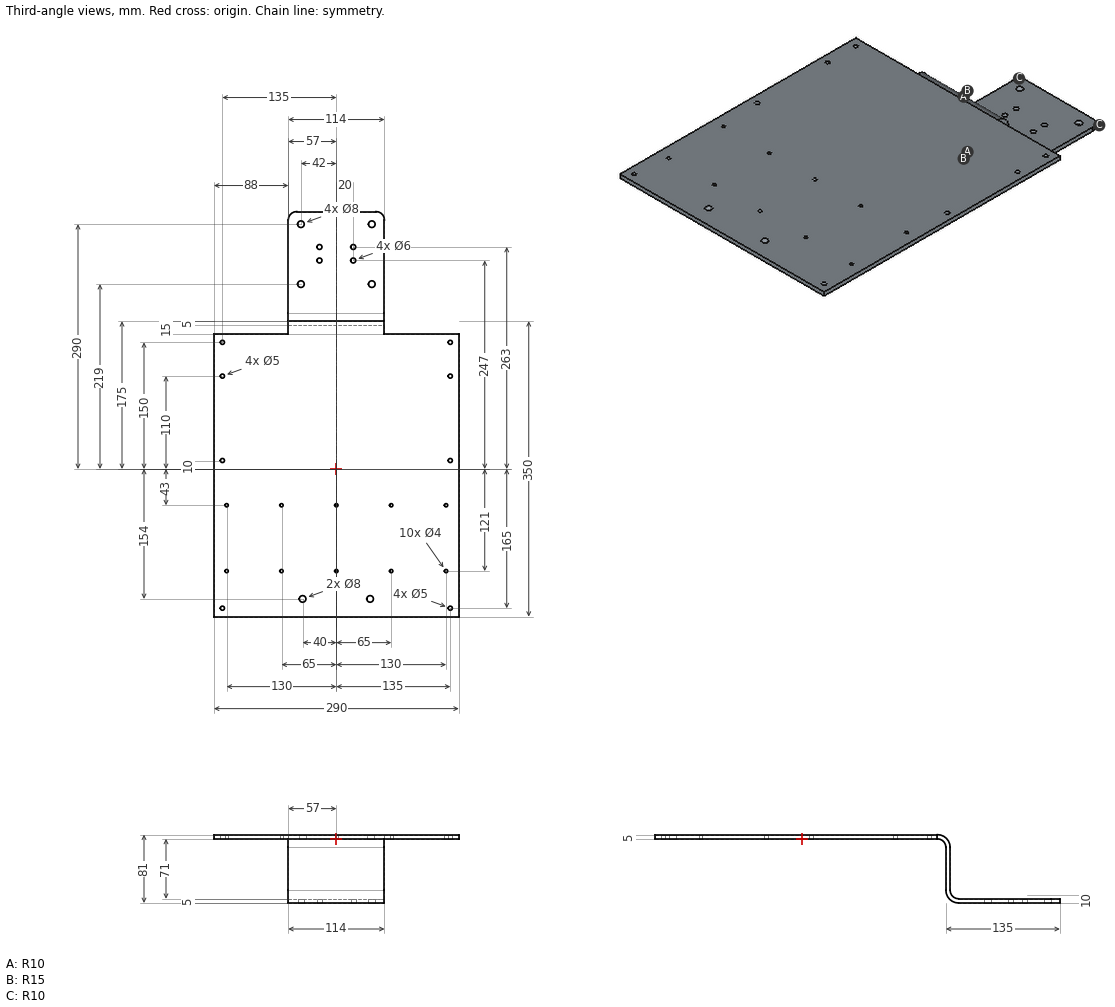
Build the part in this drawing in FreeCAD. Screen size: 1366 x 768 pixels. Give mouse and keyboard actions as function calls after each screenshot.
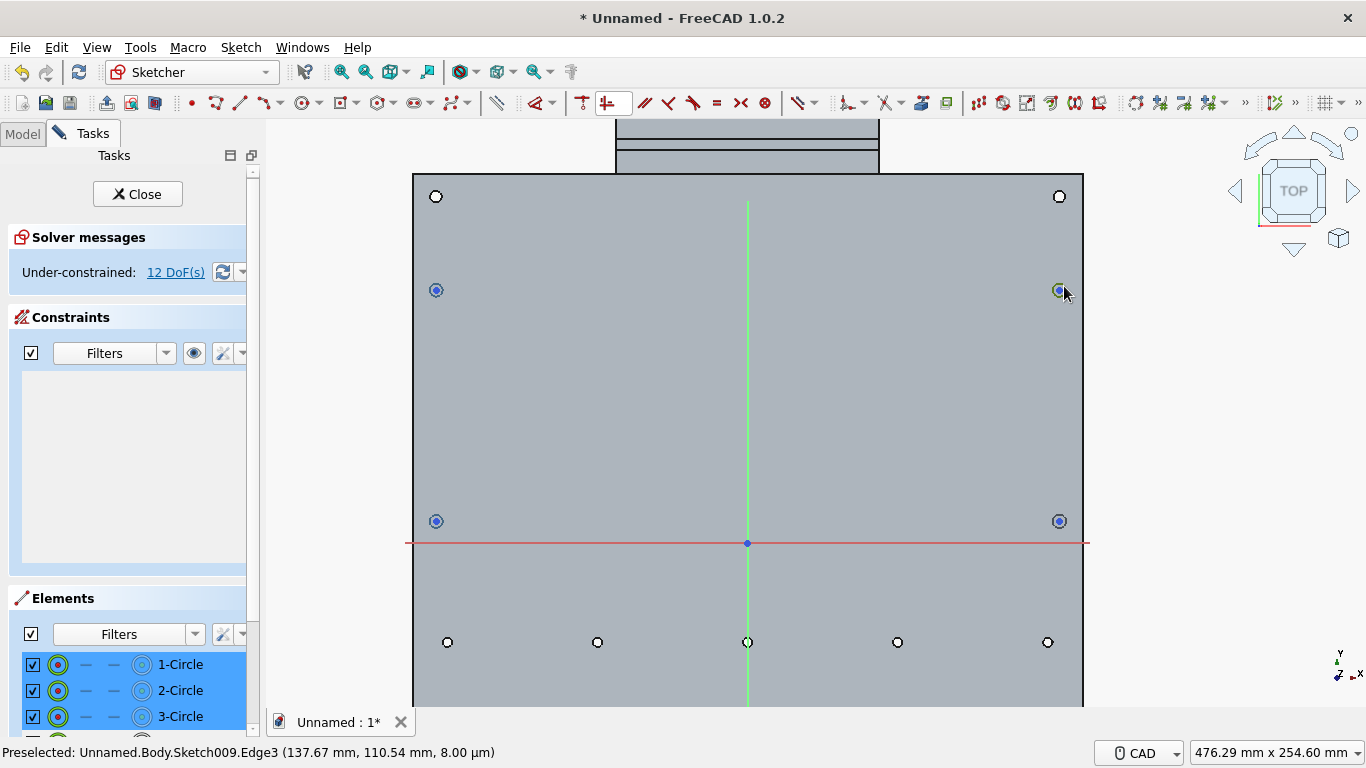
scroll(1064, 517, up, 4)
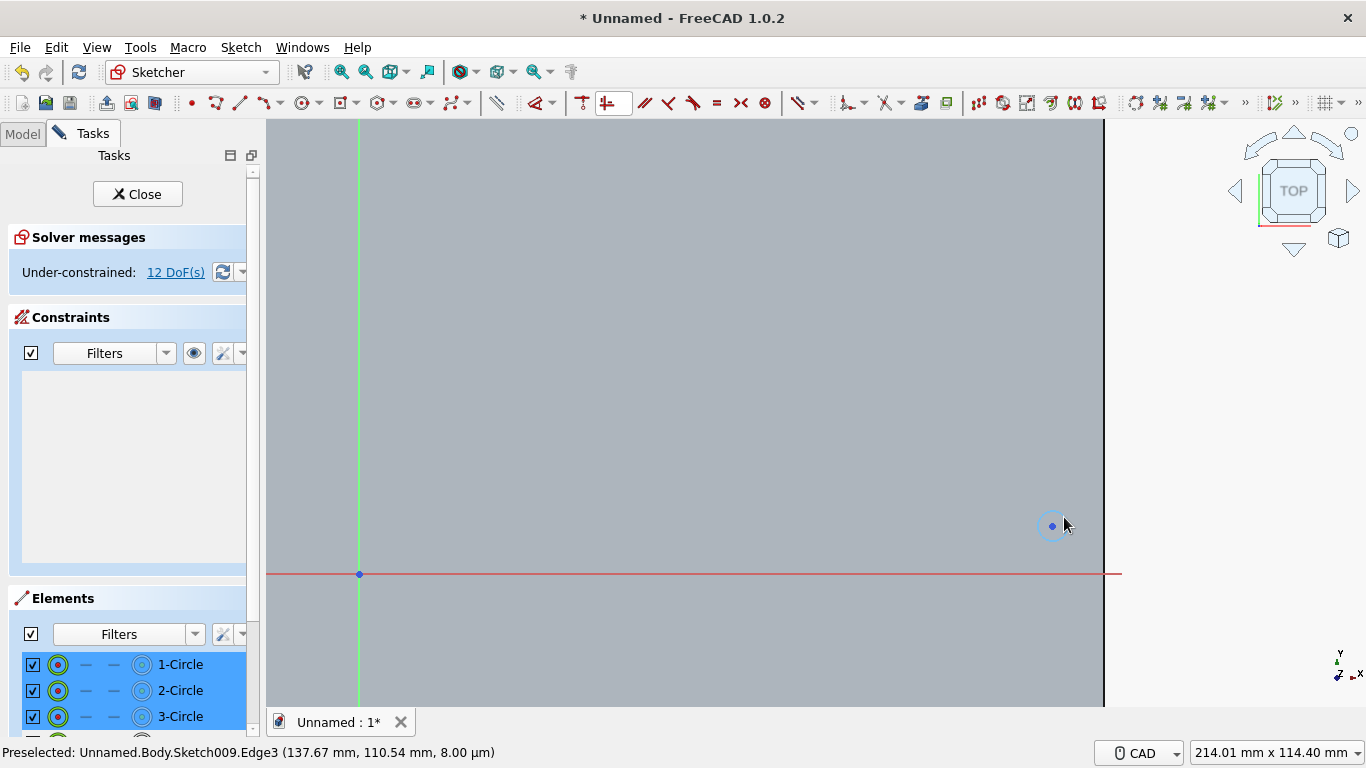
click(1064, 515)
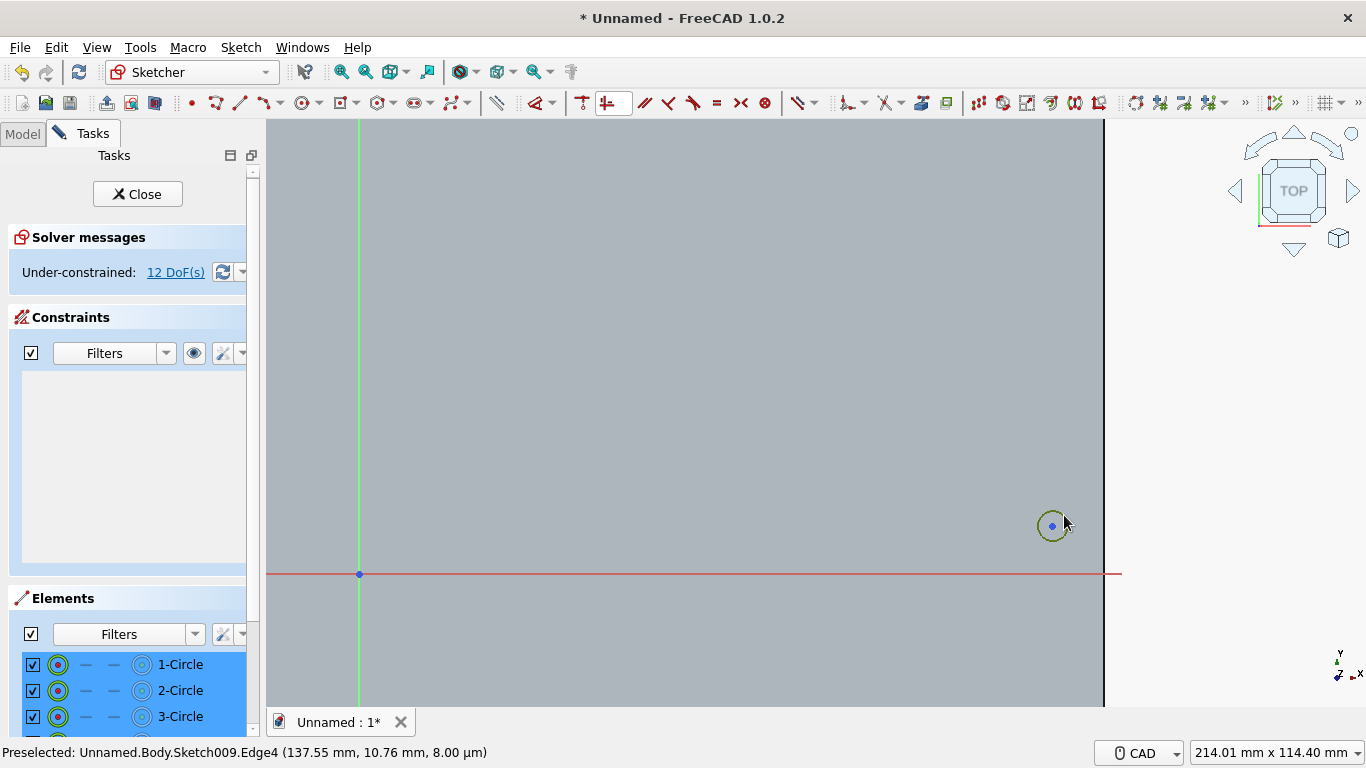
click(718, 104)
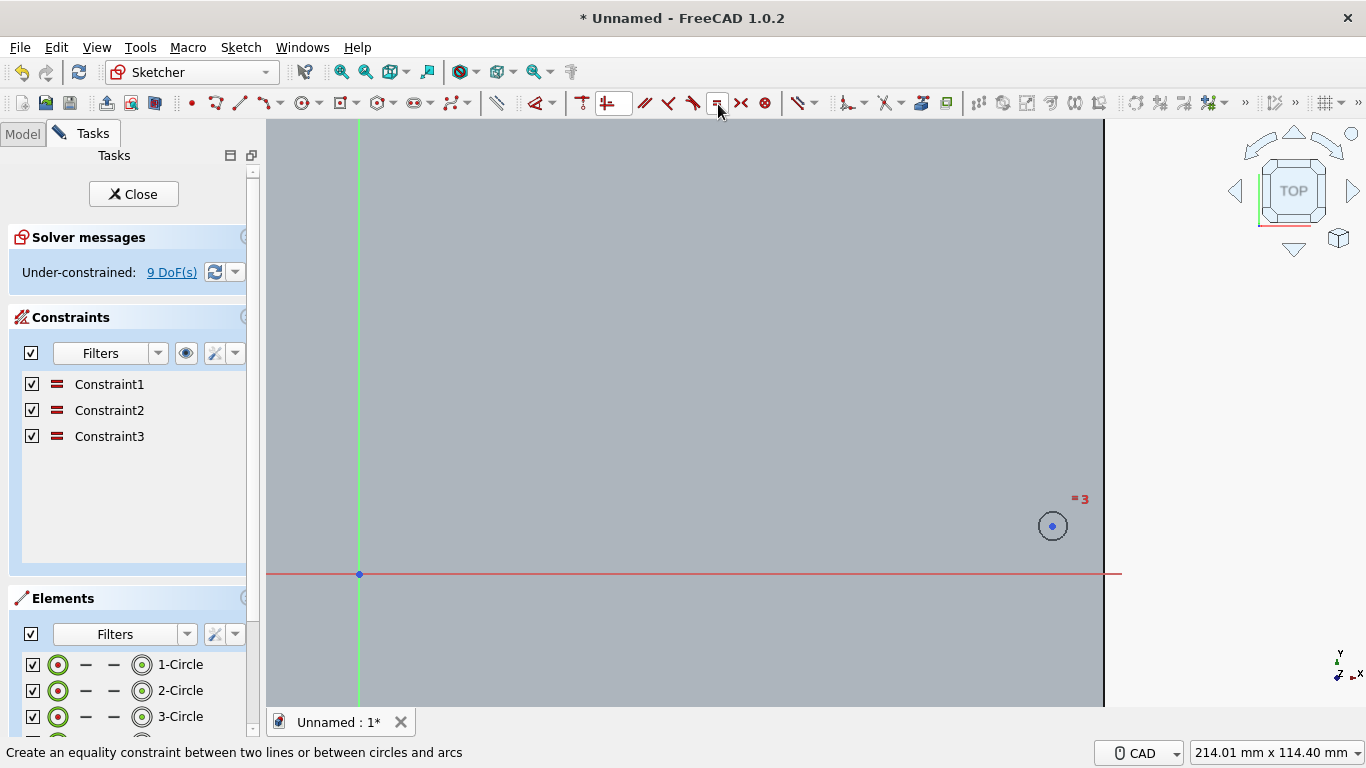
scroll(1064, 517, down, 4)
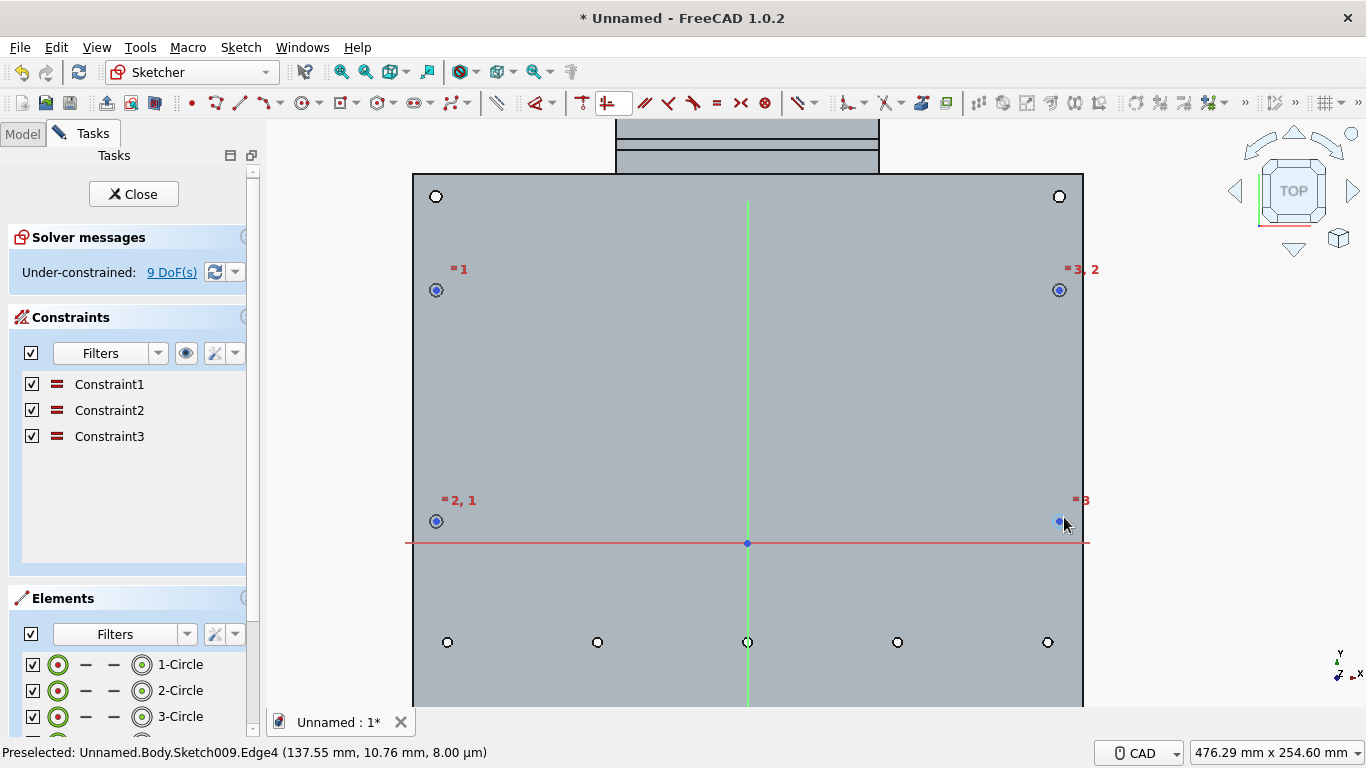
click(436, 290)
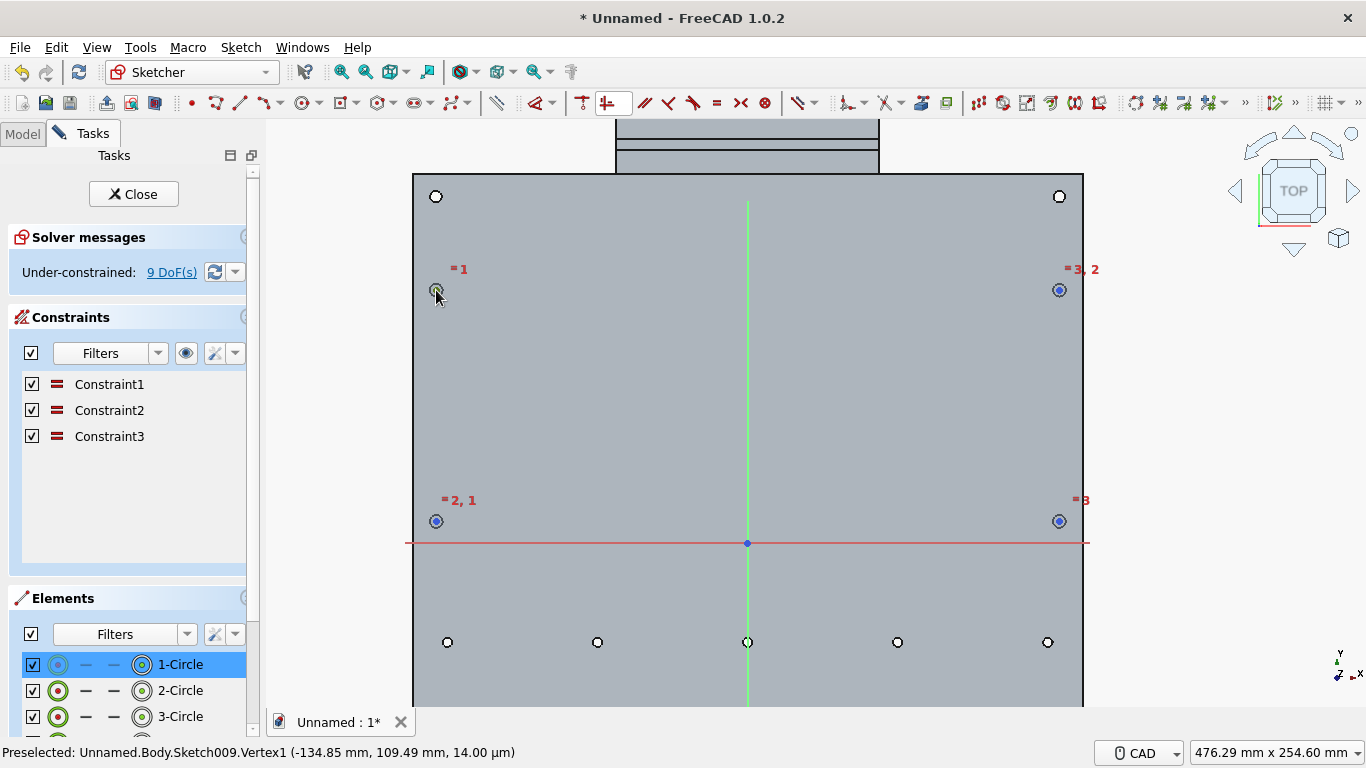
click(1059, 290)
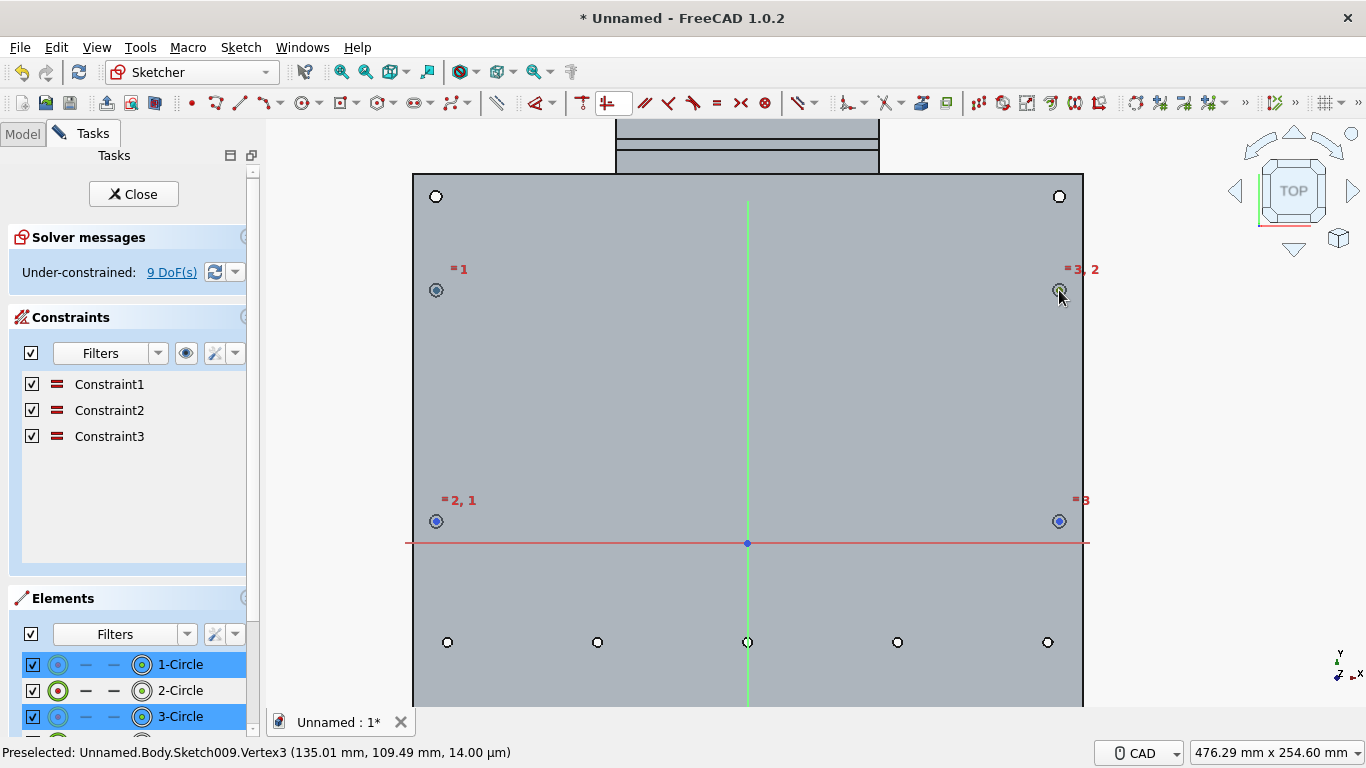
click(748, 641)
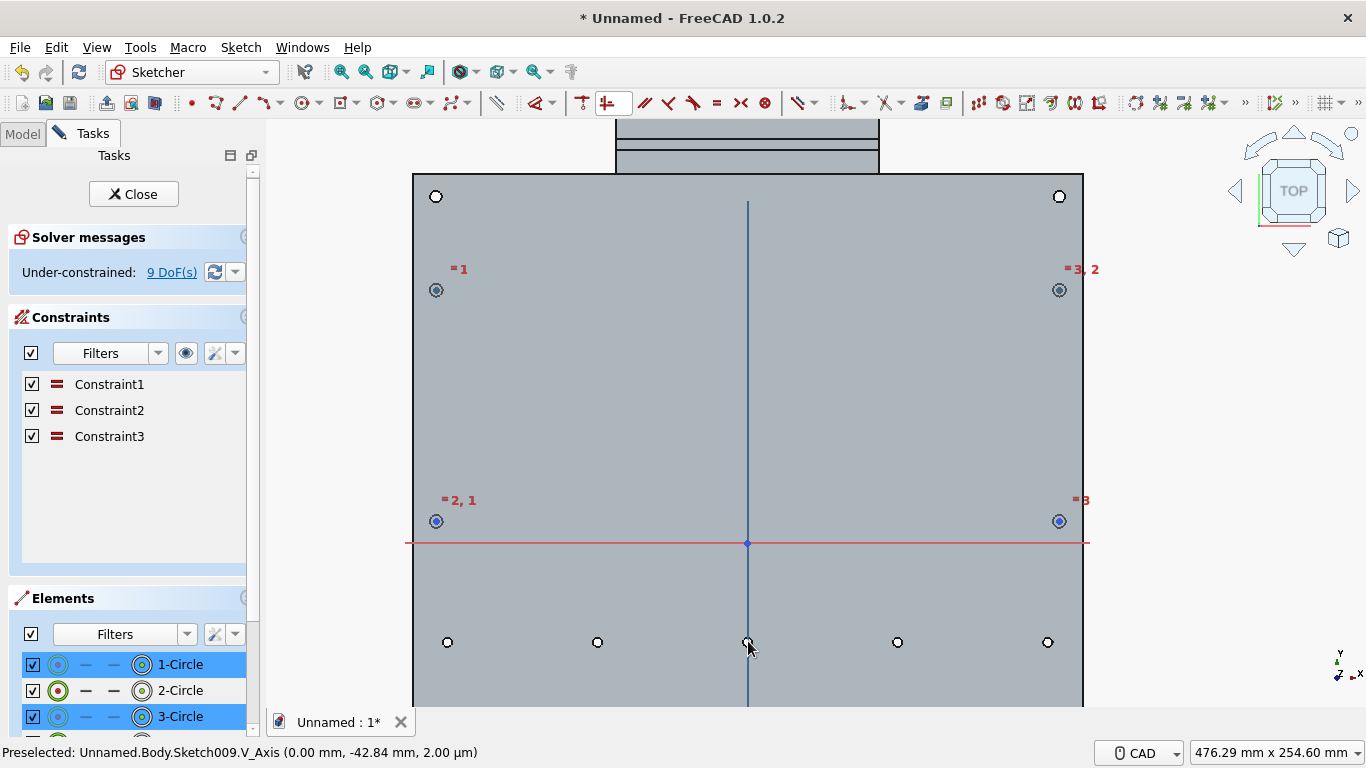
key(s)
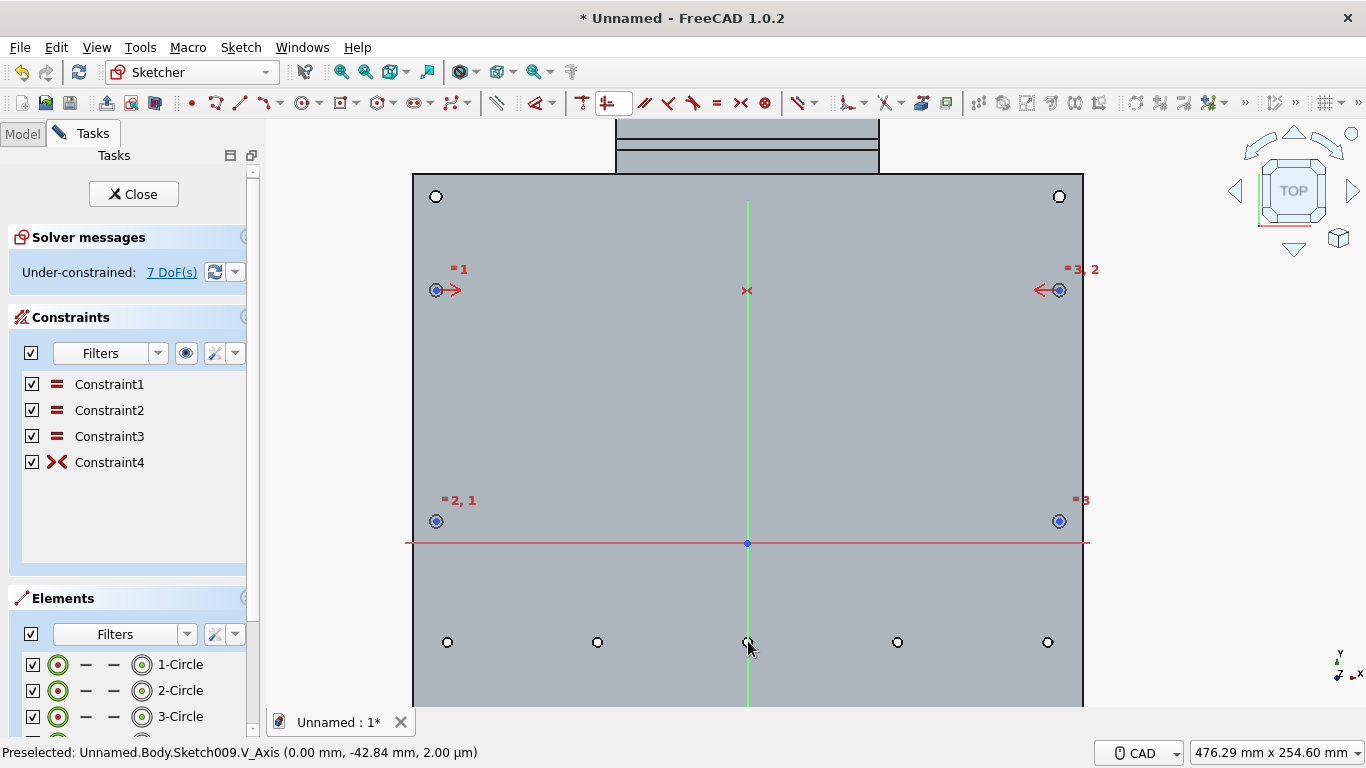
click(436, 521)